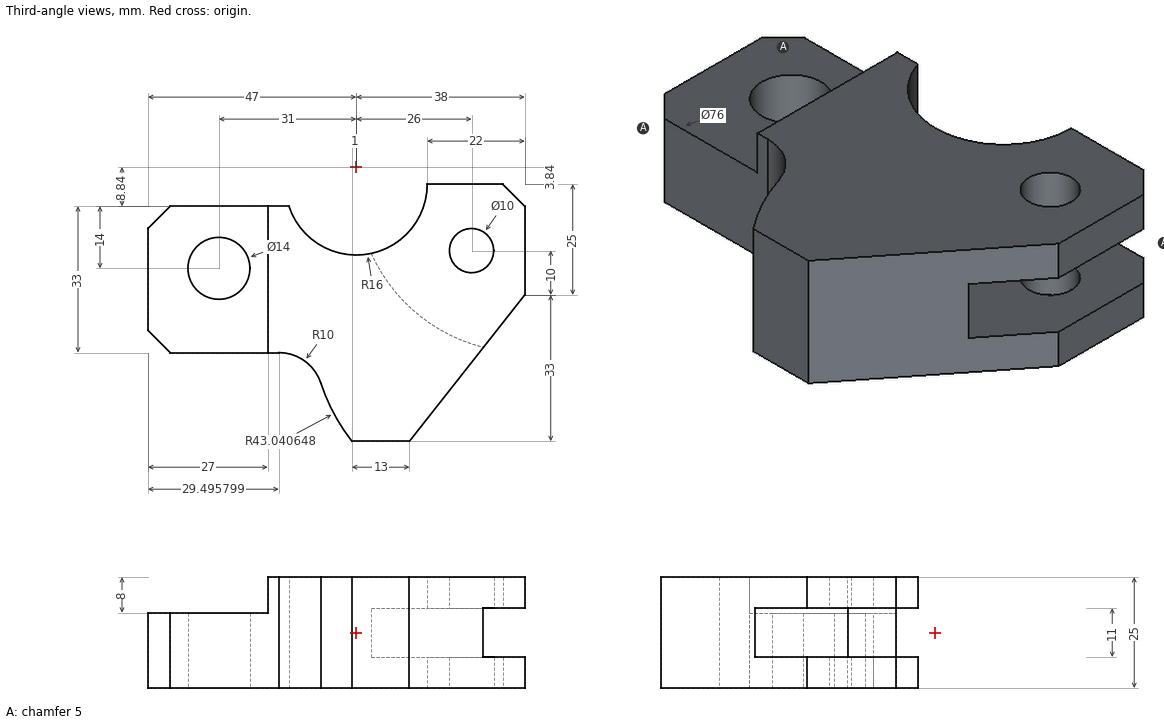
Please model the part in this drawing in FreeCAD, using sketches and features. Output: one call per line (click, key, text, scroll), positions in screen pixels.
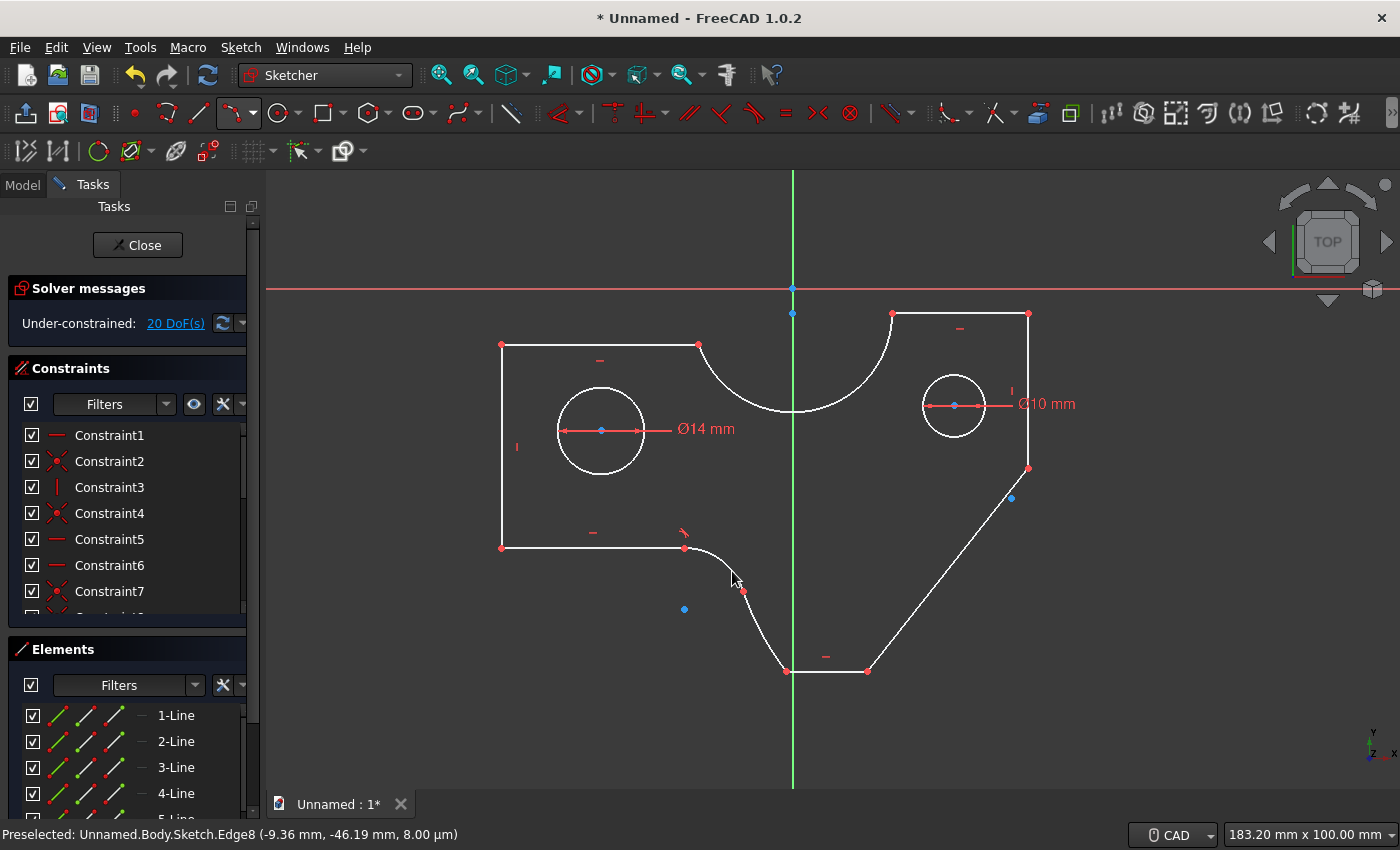
click(732, 571)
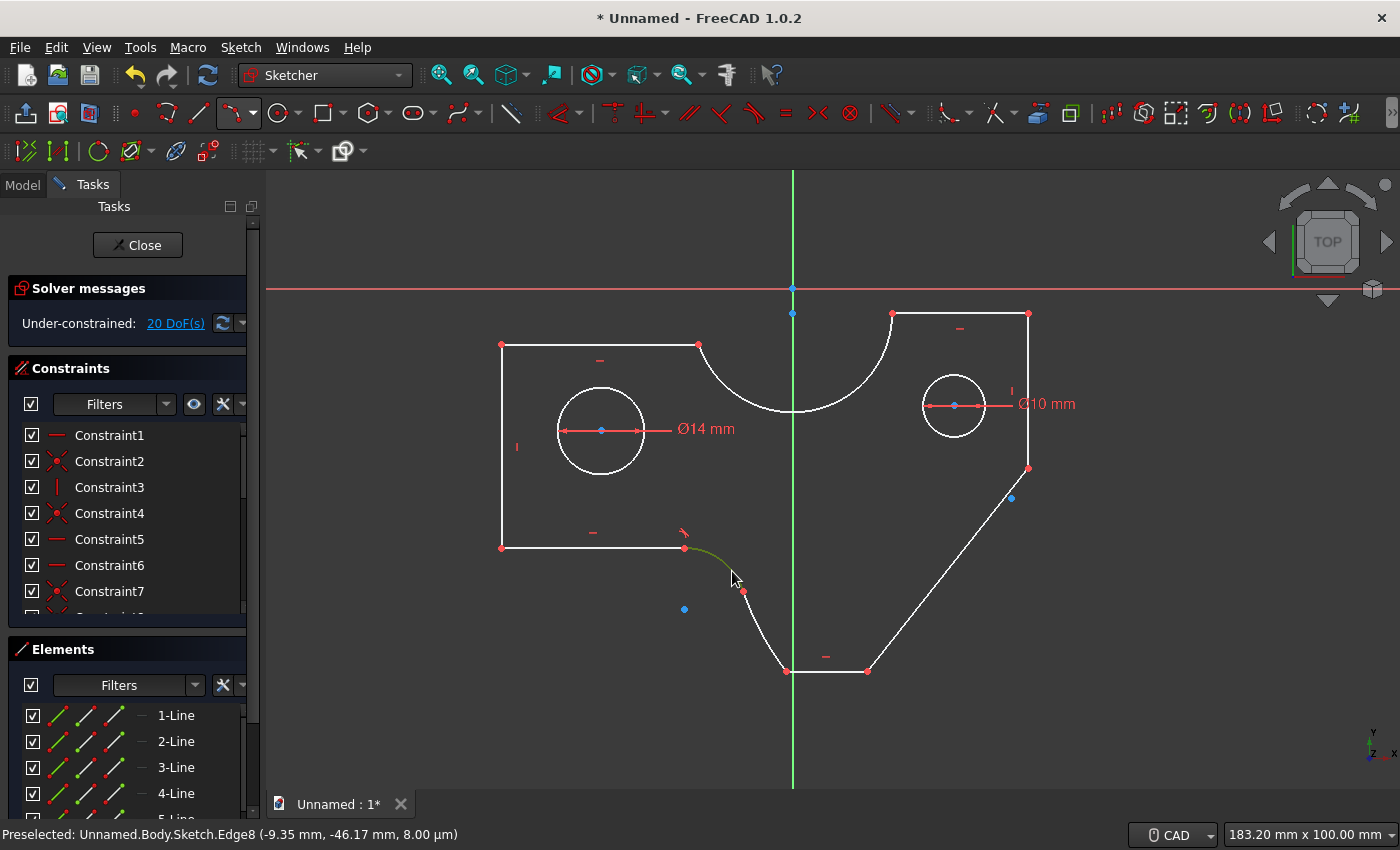
click(753, 617)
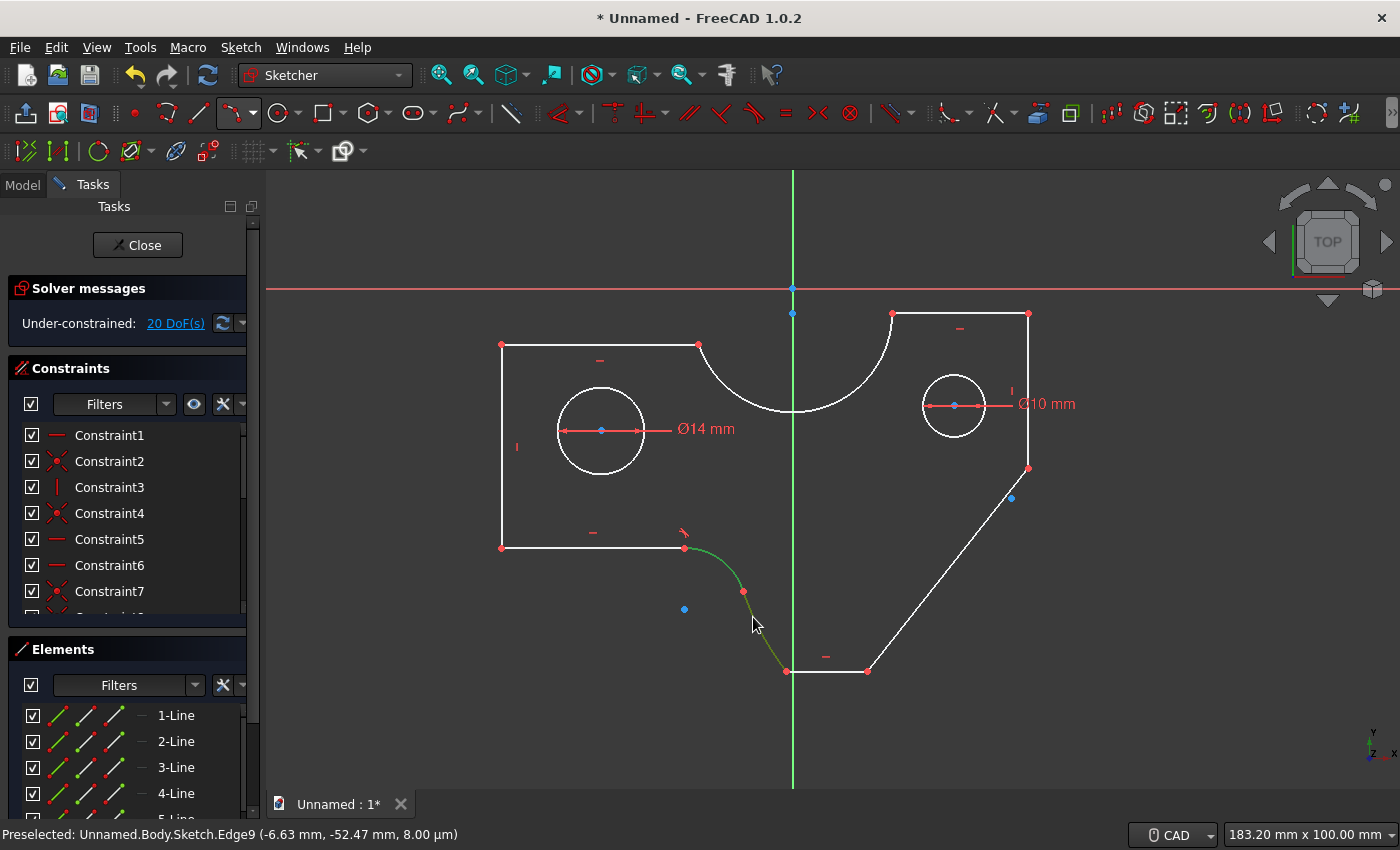
key(t)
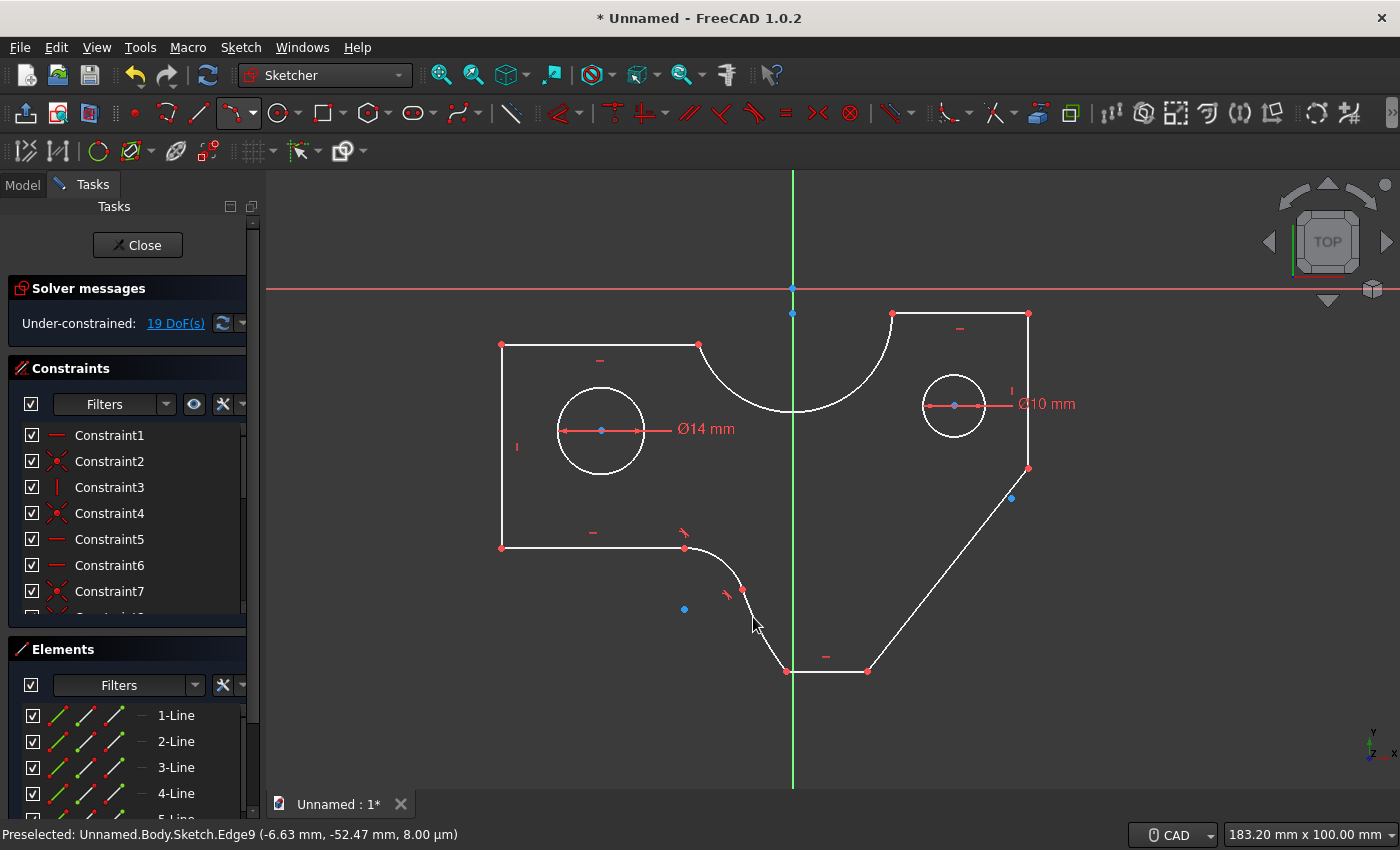
click(793, 313)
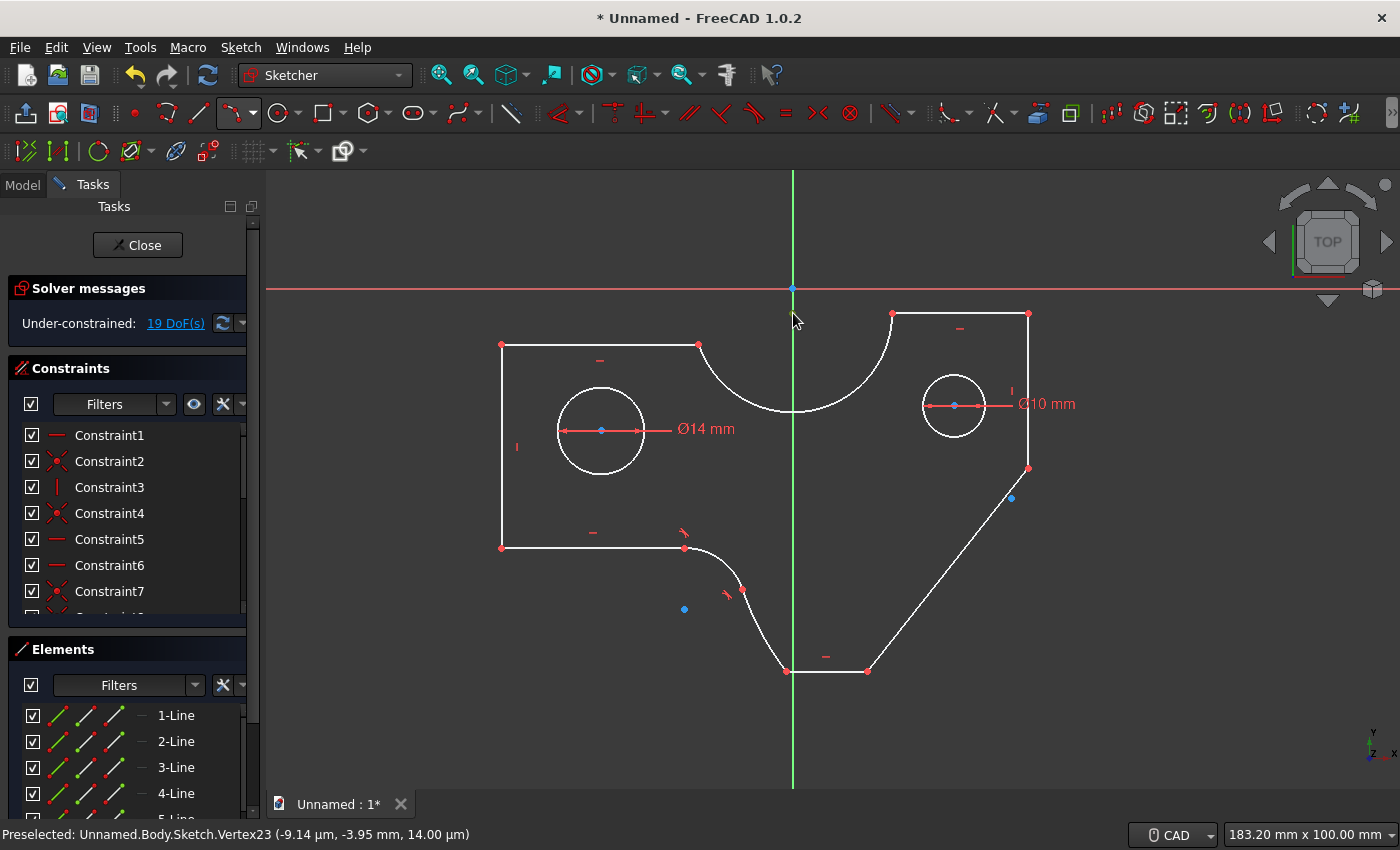
click(793, 721)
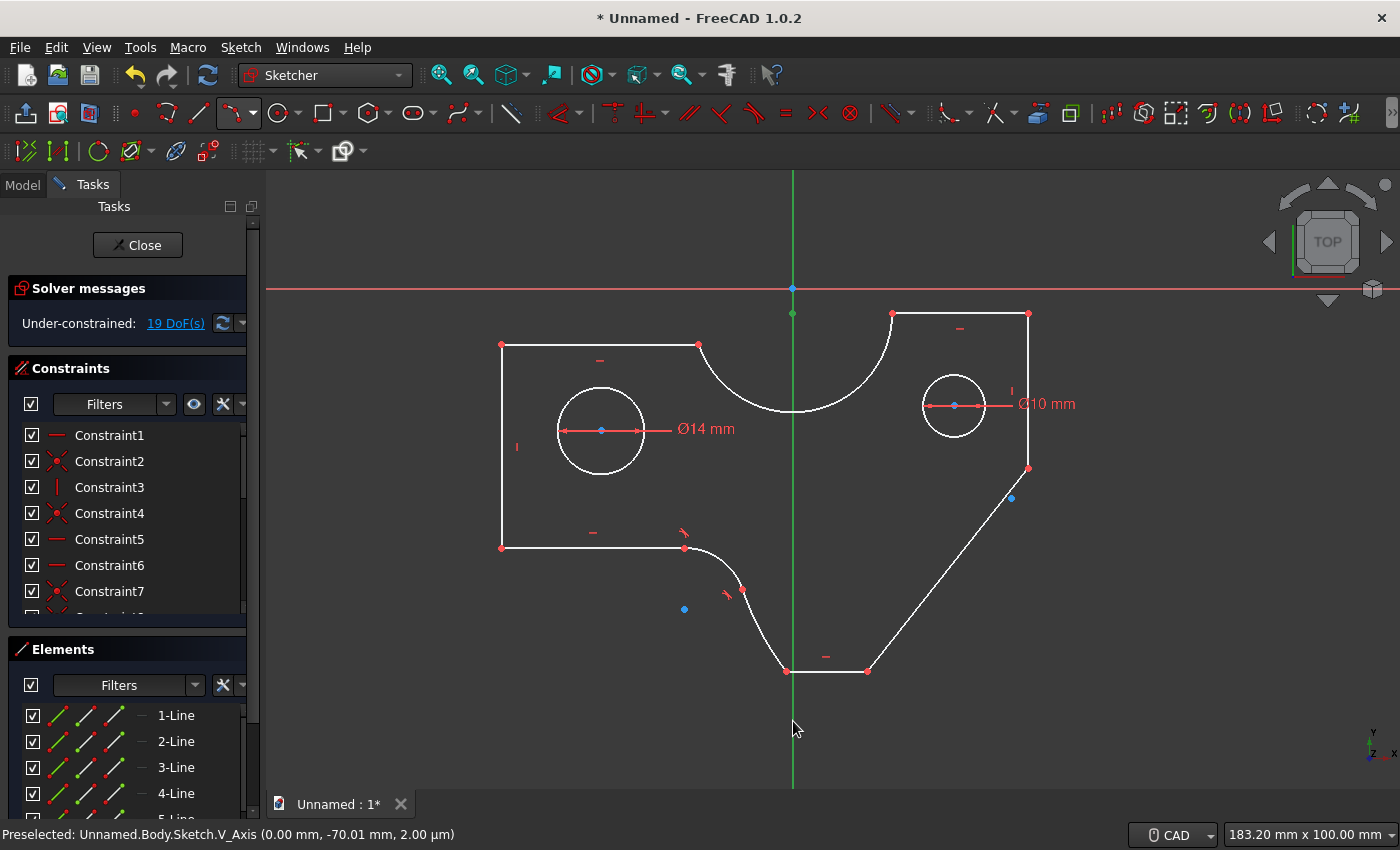
key(c)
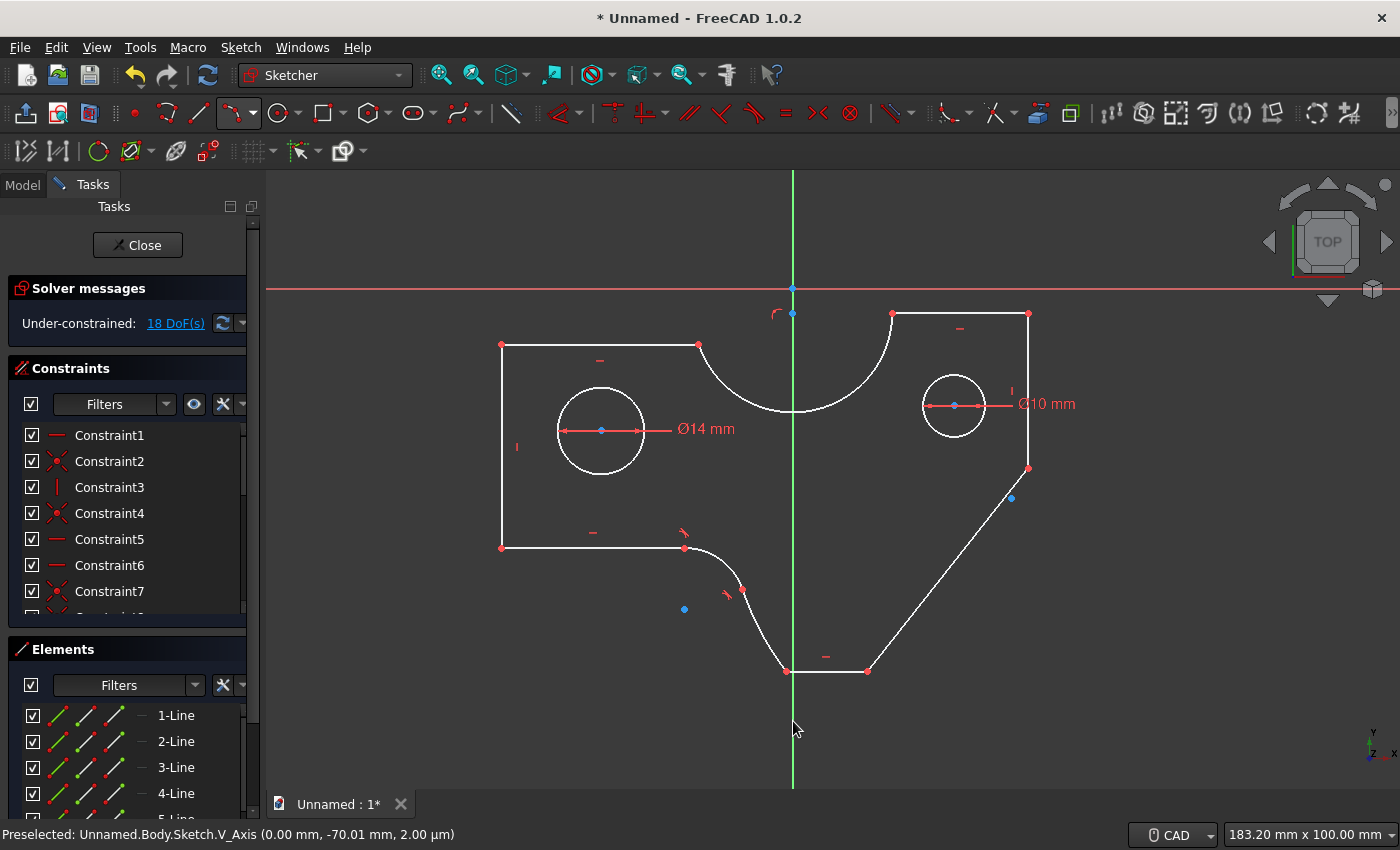
click(558, 114)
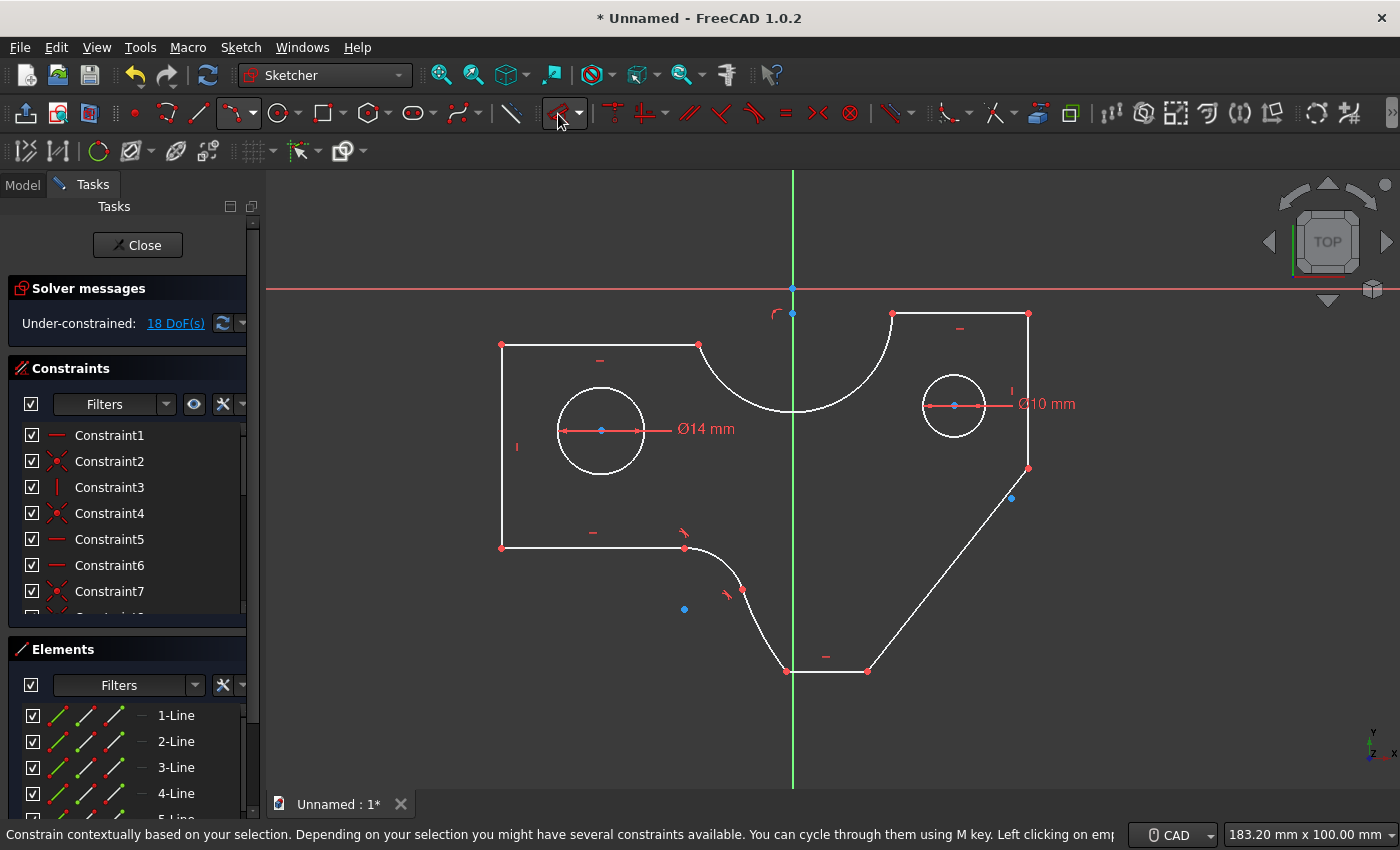
click(731, 570)
click(755, 549)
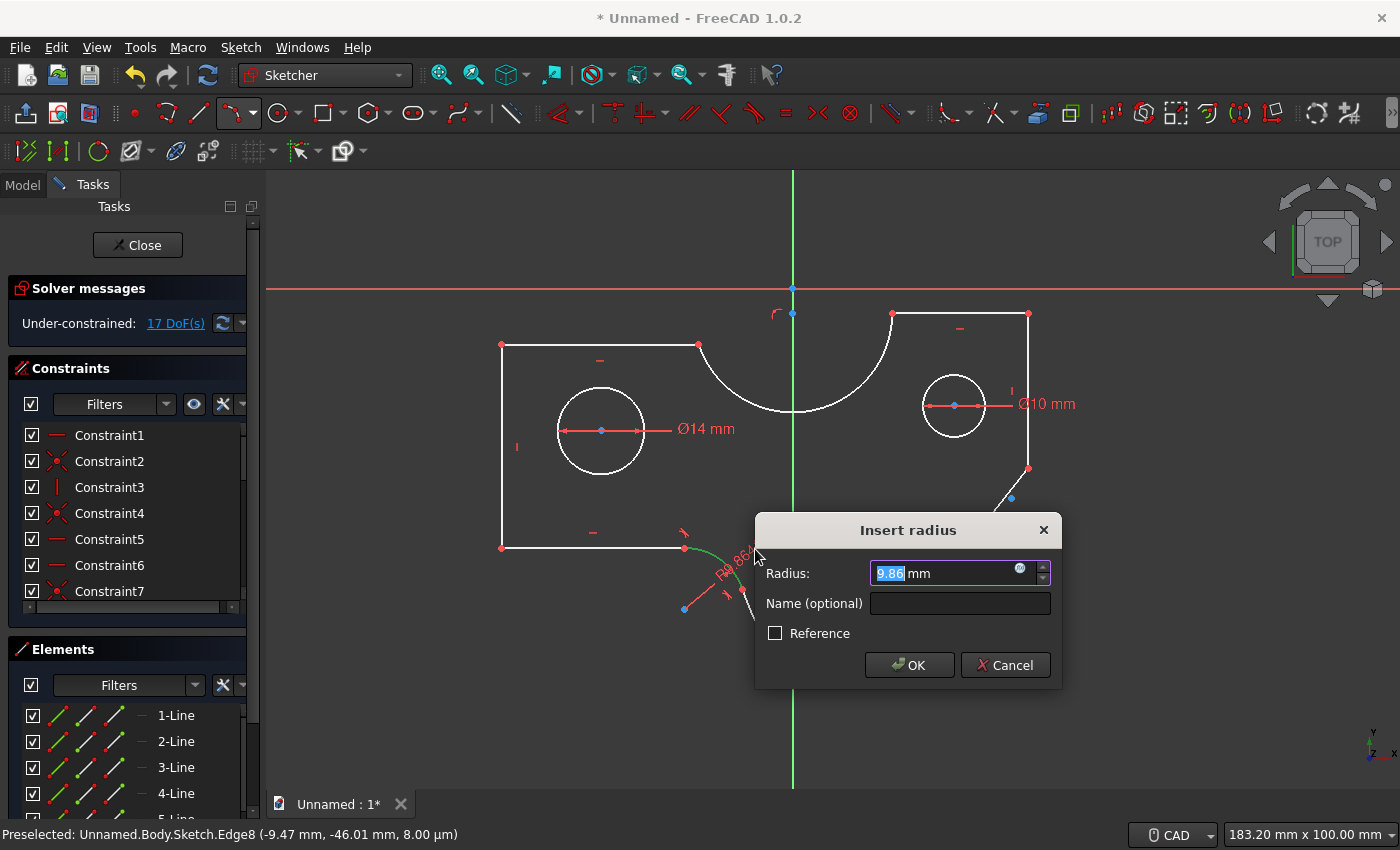
text(10)
key(Return)